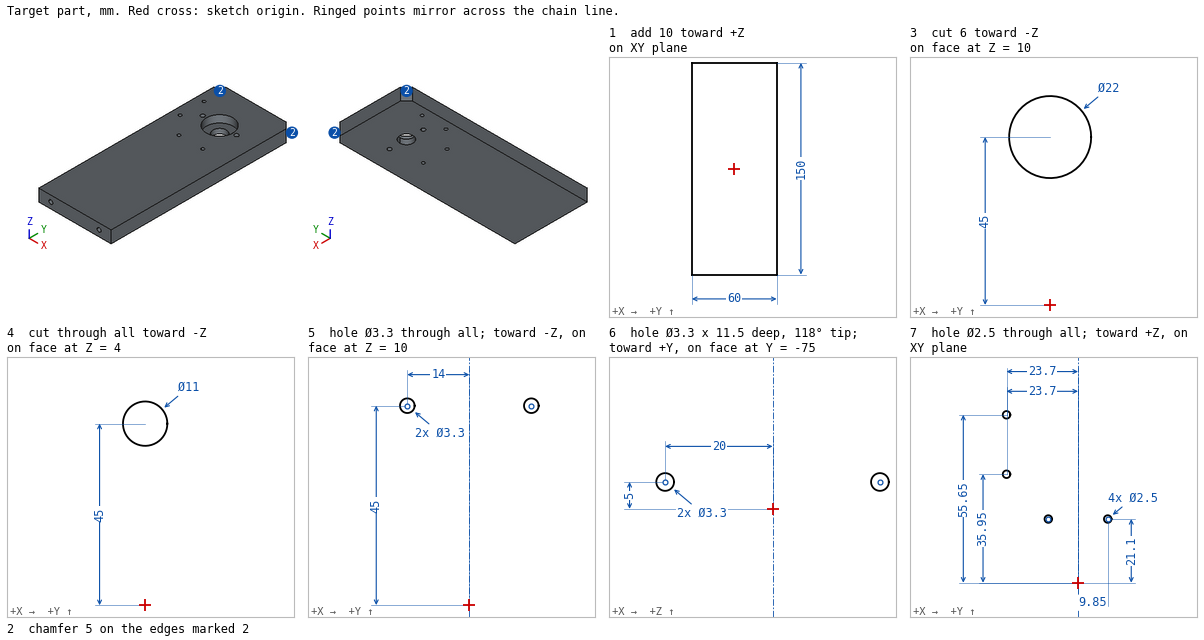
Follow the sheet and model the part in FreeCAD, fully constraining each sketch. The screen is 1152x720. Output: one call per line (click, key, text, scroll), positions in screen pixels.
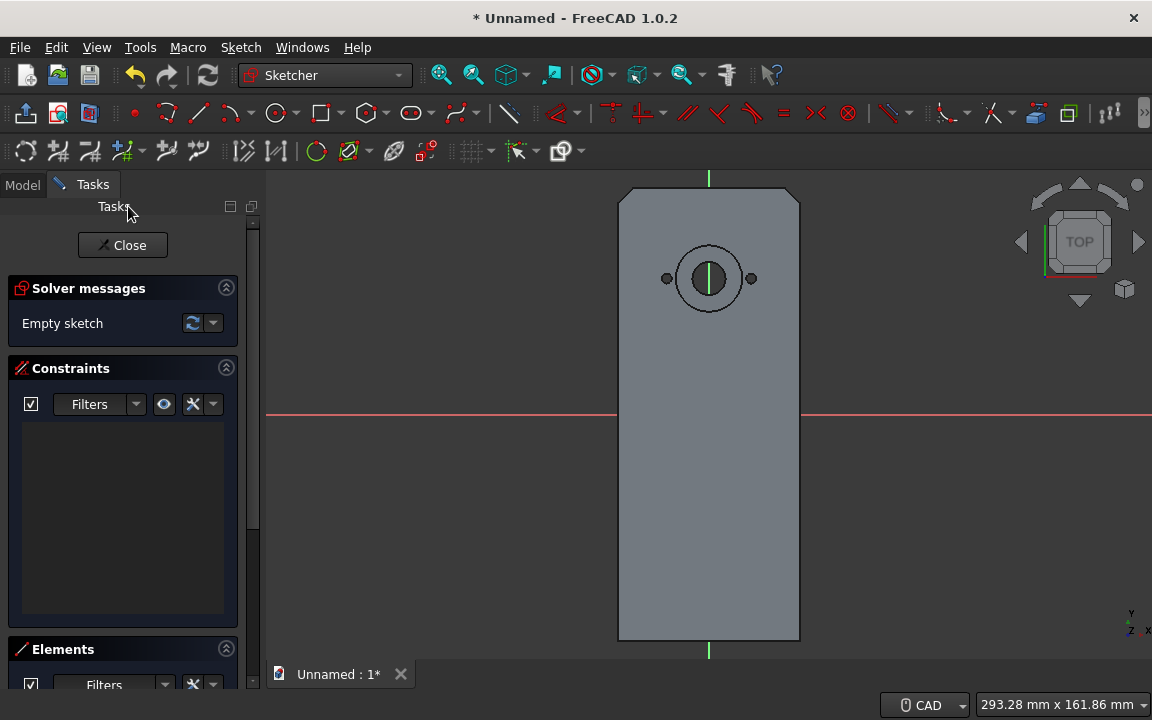
click(90, 114)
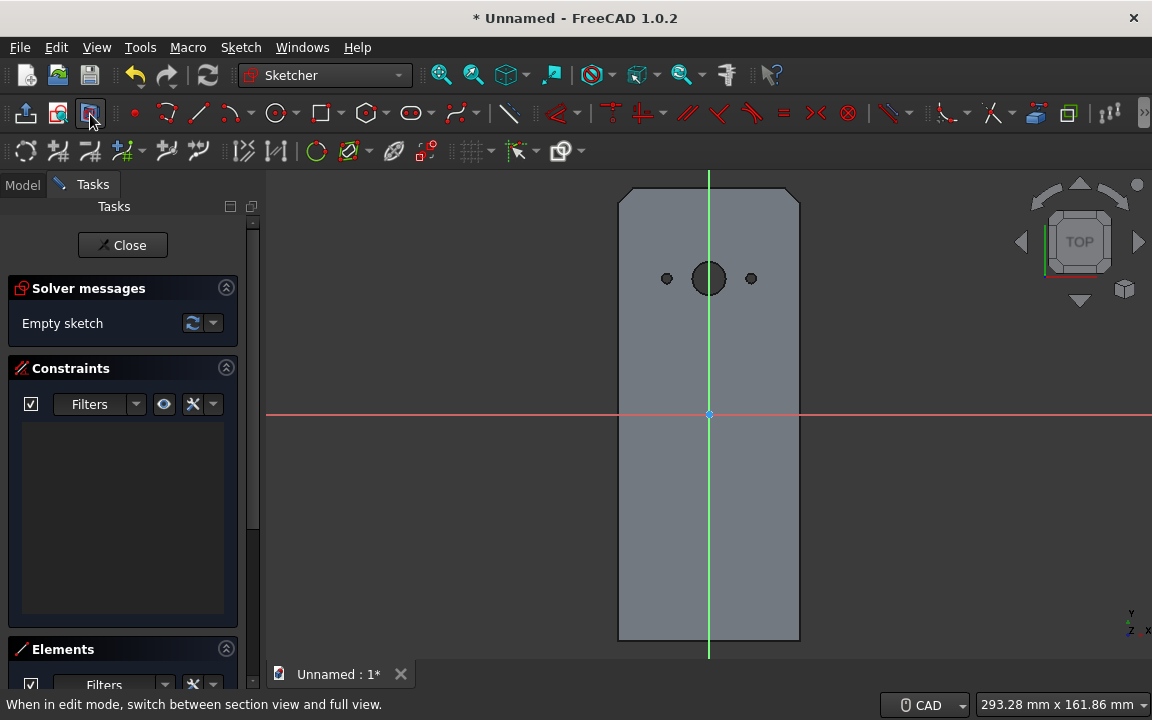
scroll(746, 224, up, 3)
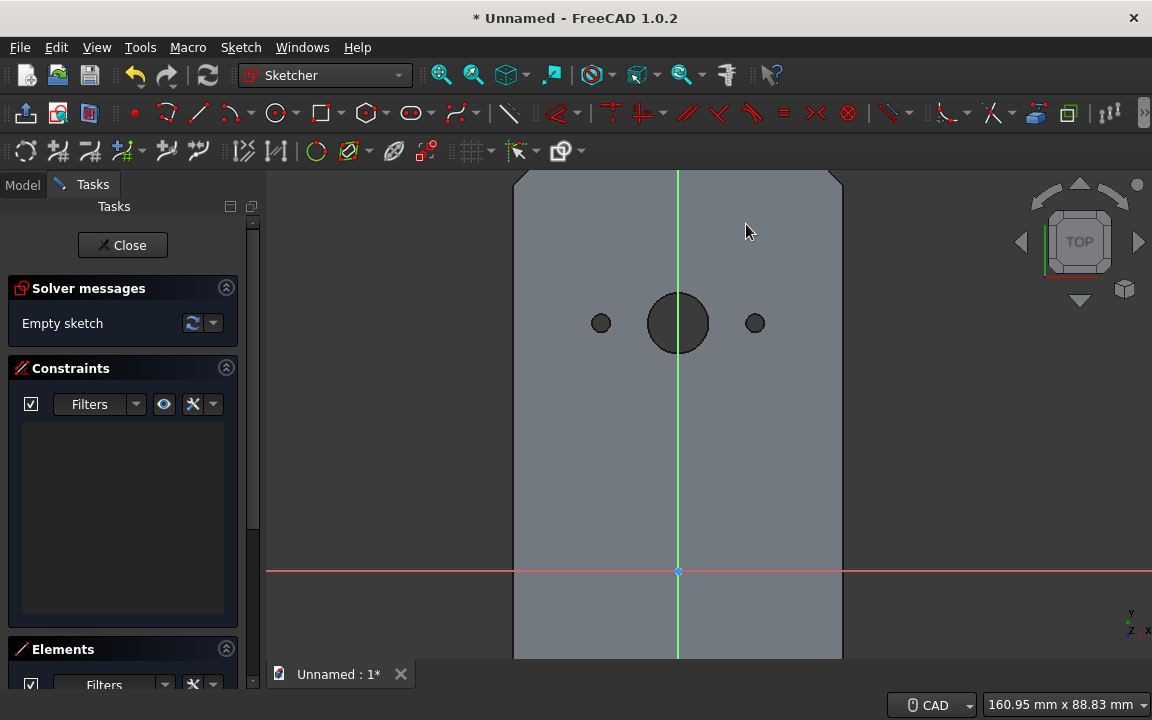
click(276, 114)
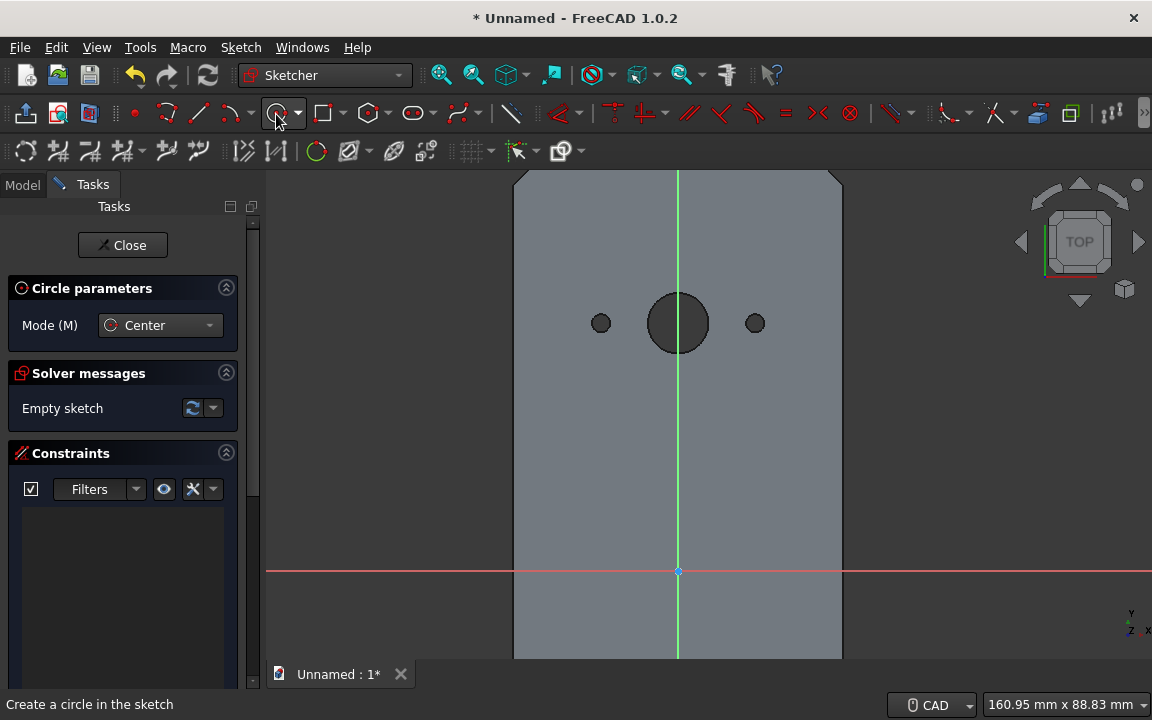
scroll(732, 455, up, 6)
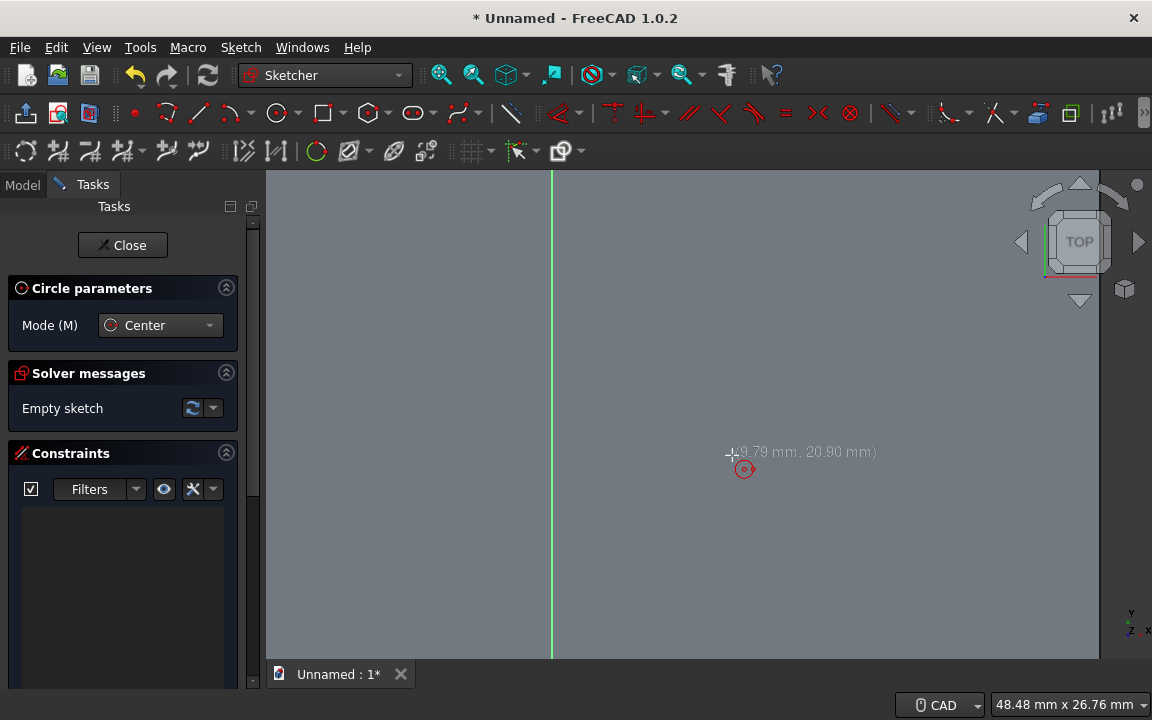
click(732, 453)
click(748, 437)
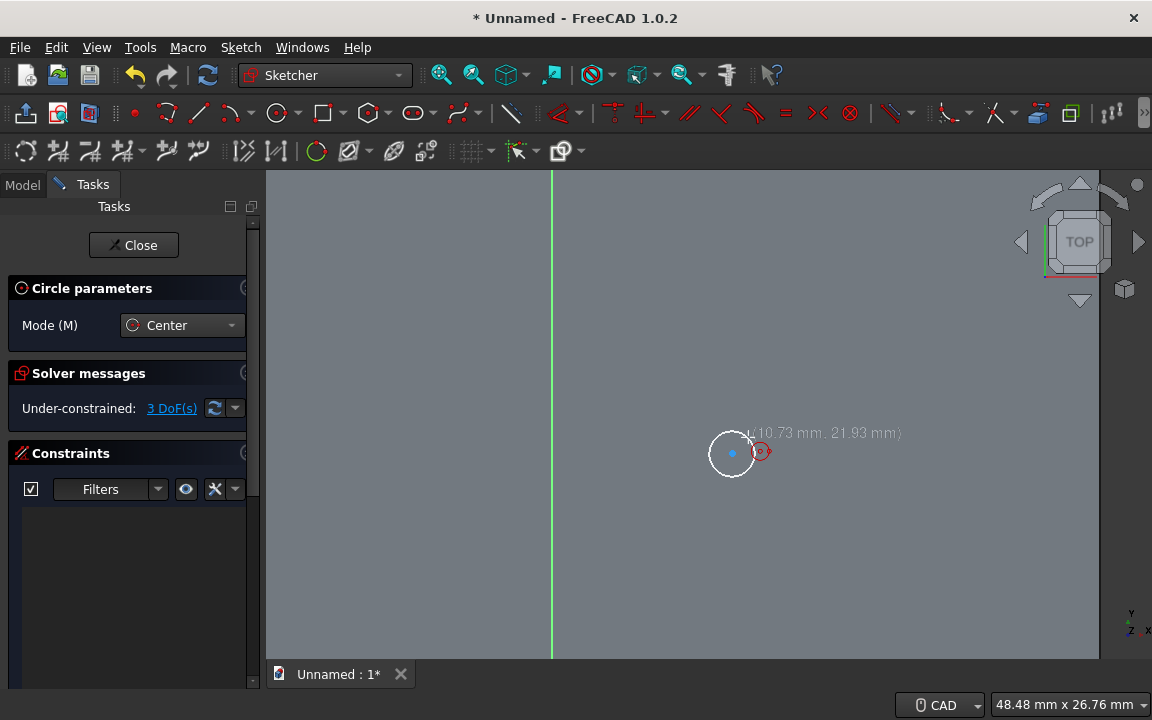
click(372, 453)
click(388, 437)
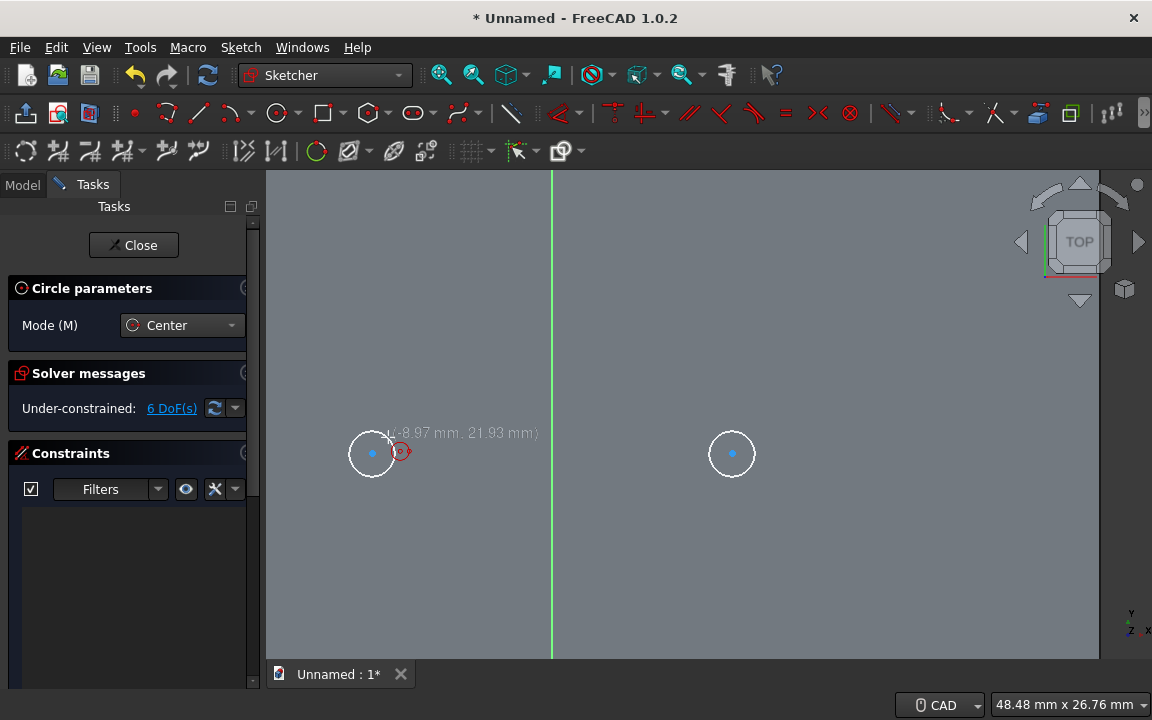
scroll(733, 456, down, 6)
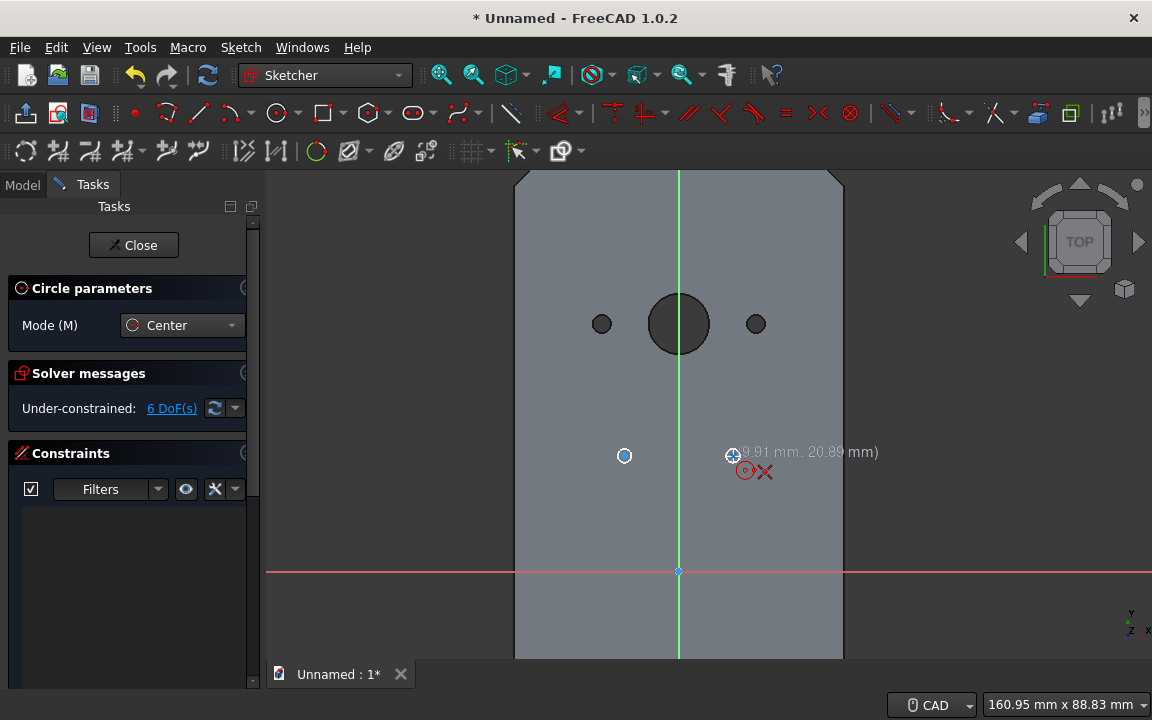
scroll(548, 374, up, 6)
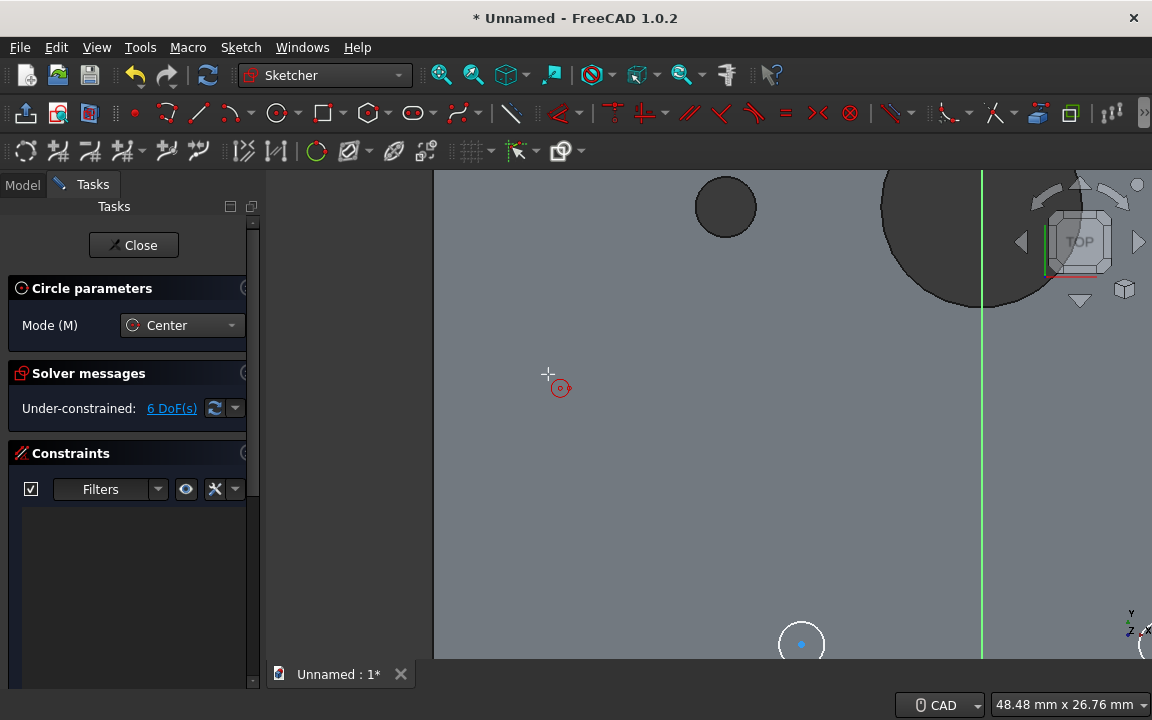
click(549, 372)
click(565, 356)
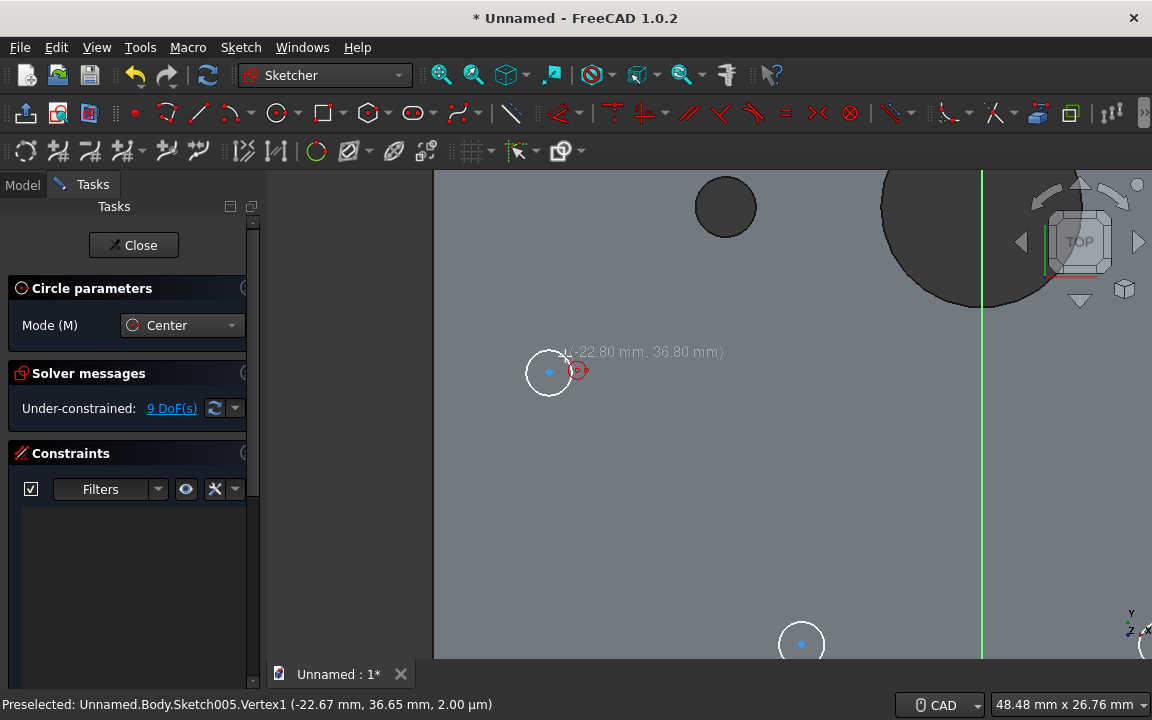
scroll(548, 374, down, 6)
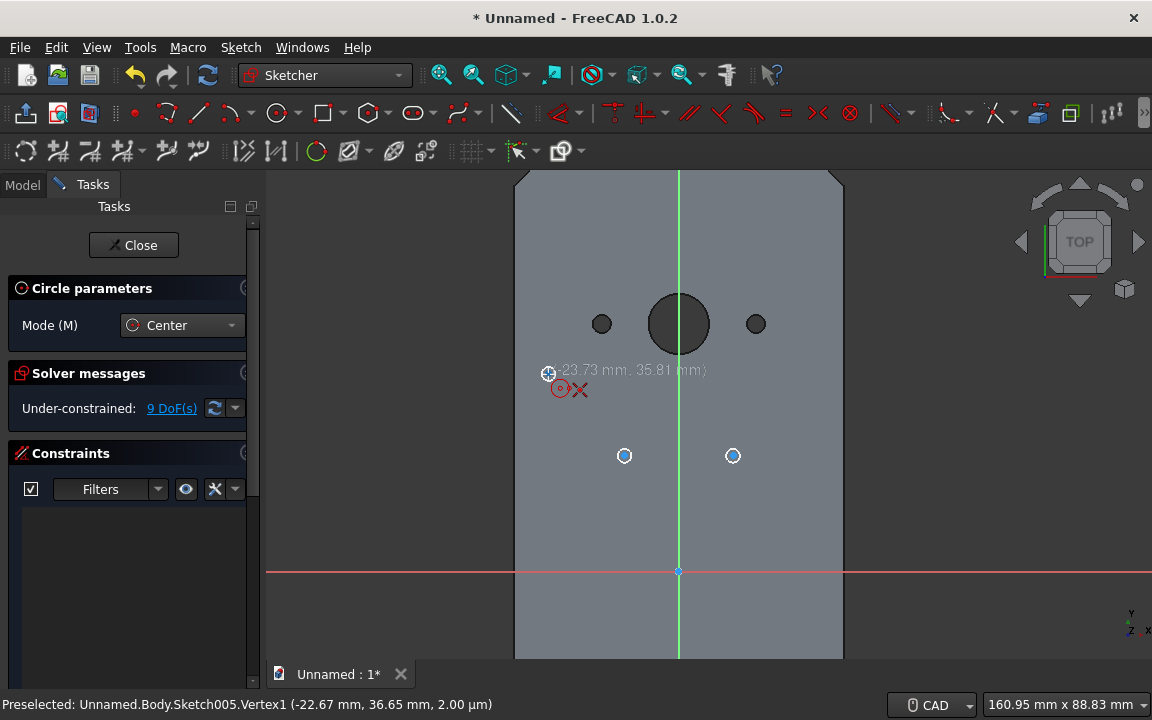
scroll(548, 265, up, 6)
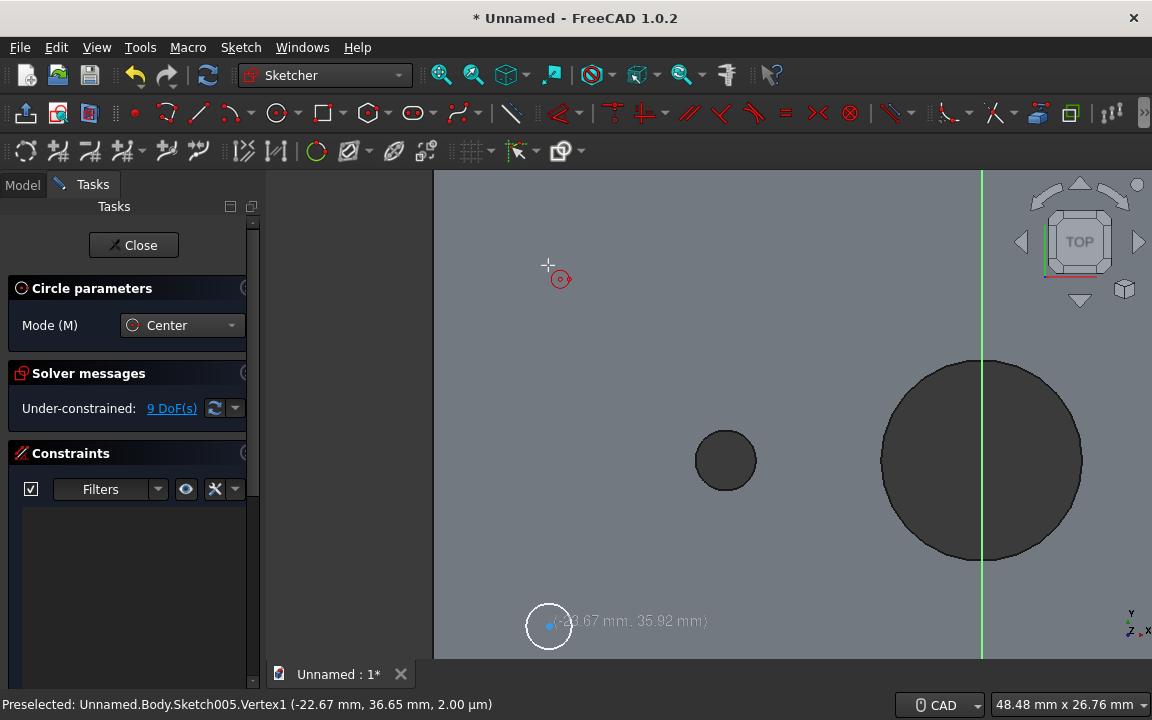
click(549, 266)
click(565, 250)
key(Escape)